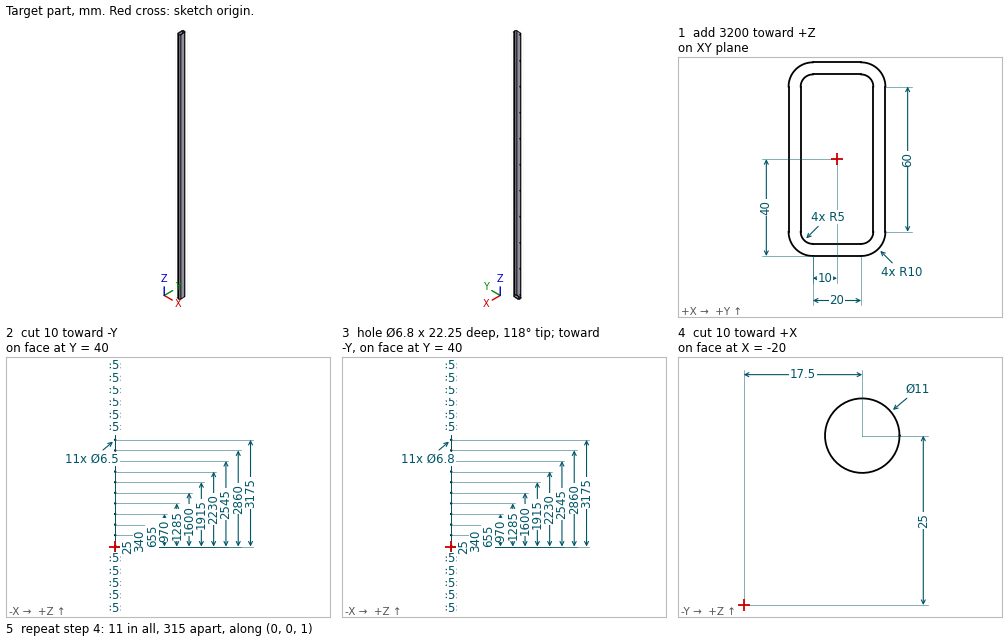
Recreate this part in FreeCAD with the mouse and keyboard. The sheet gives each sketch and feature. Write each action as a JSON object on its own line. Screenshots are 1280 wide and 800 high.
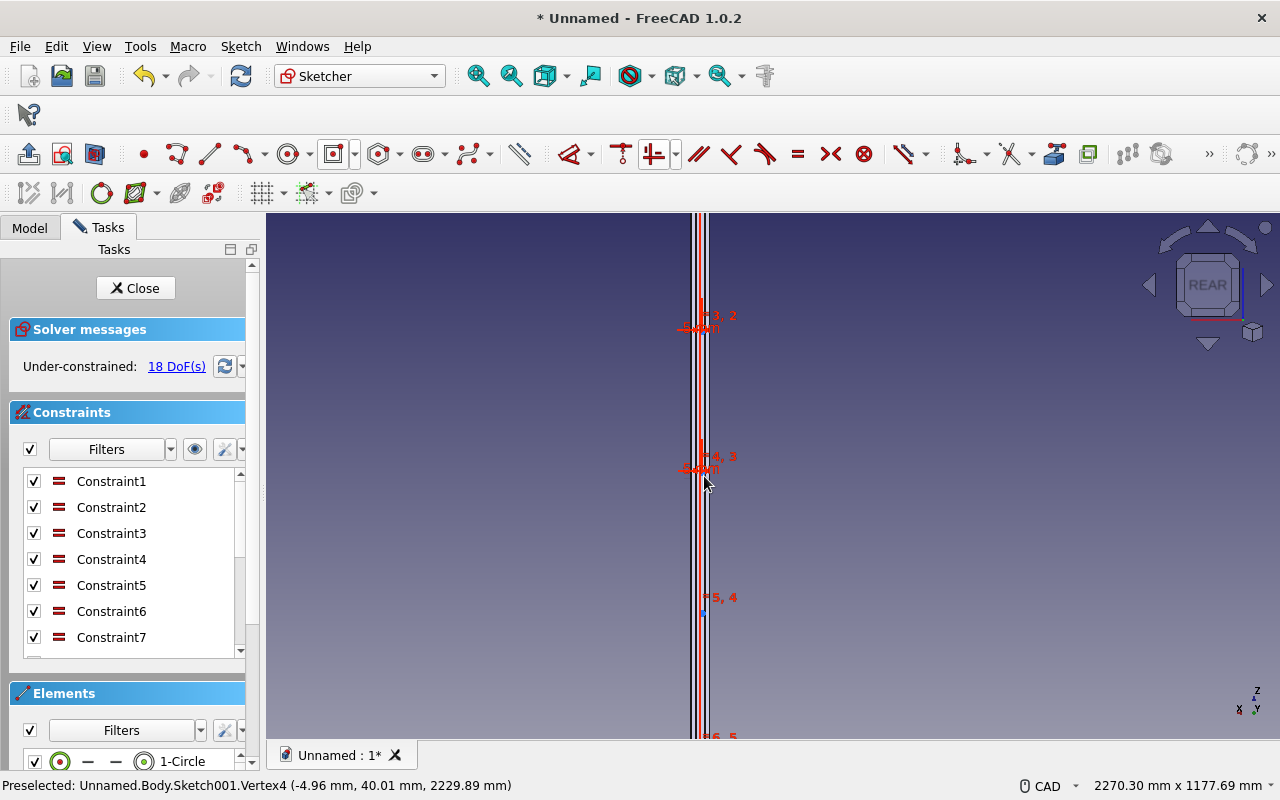
{"action": "scroll", "coordinate": [705, 383], "scroll_direction": "down", "scroll_amount": 7}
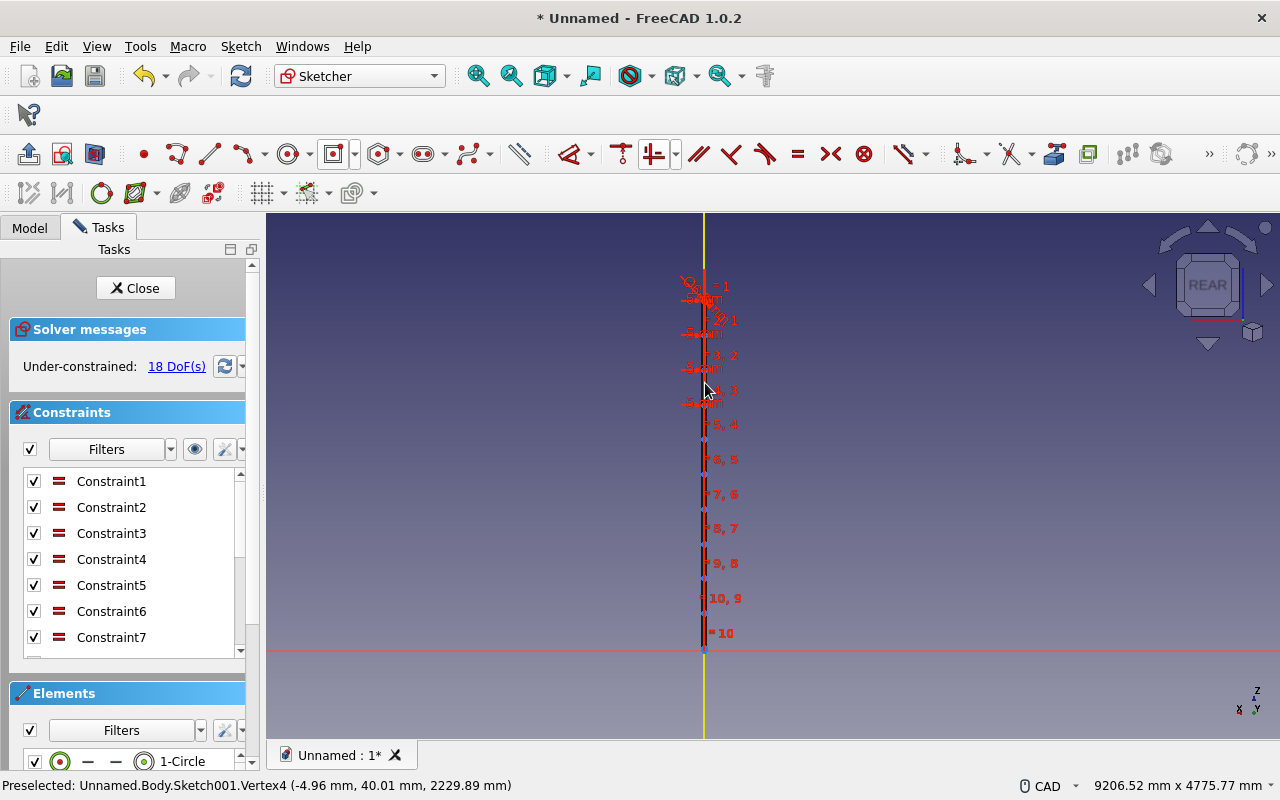
{"action": "scroll", "coordinate": [705, 440], "scroll_direction": "up", "scroll_amount": 22}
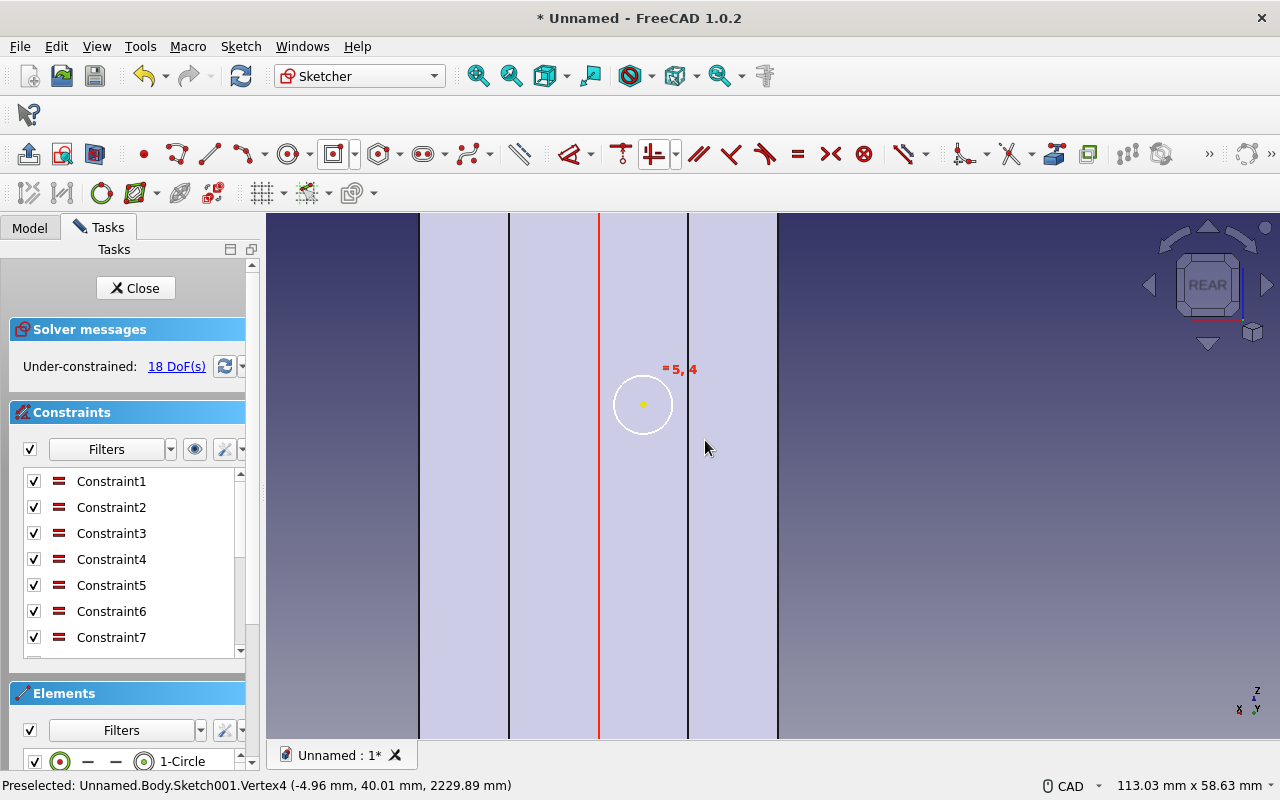
{"action": "left_click", "coordinate": [643, 405]}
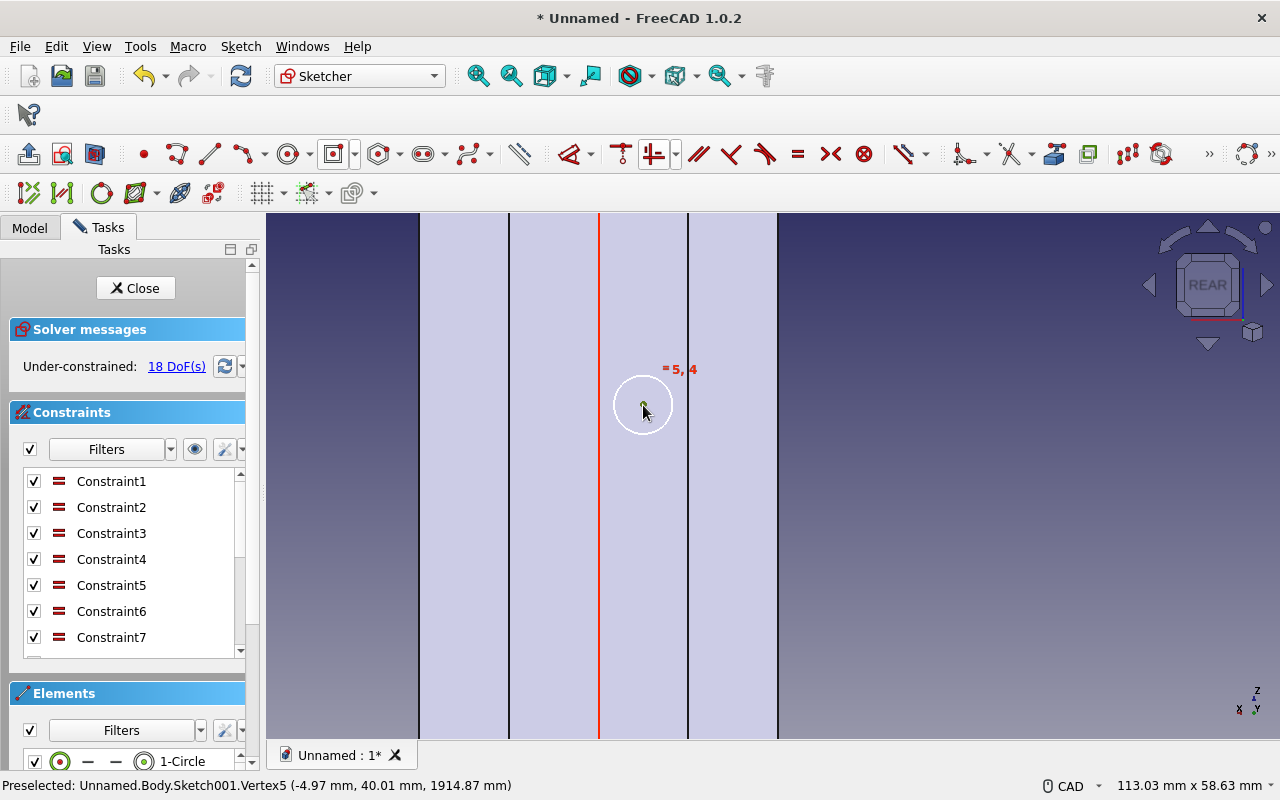
{"action": "key", "text": "l"}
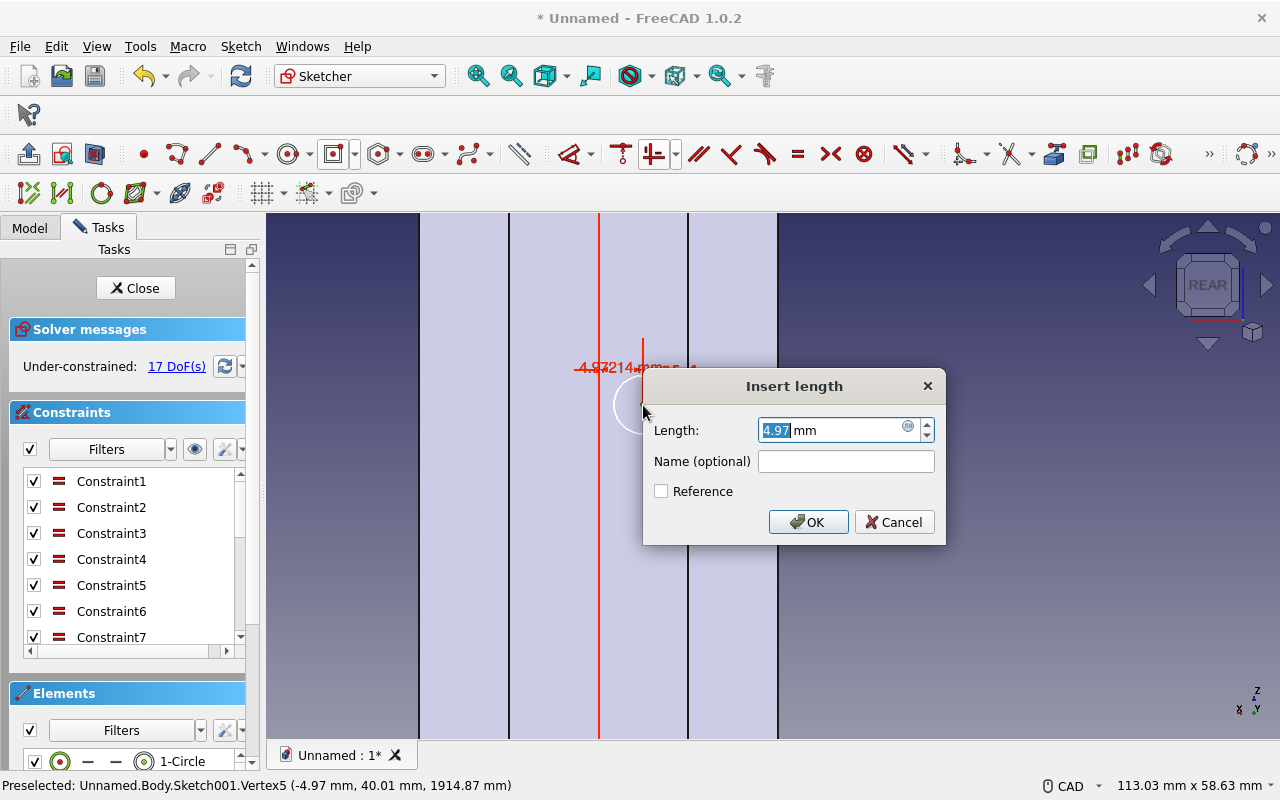
{"action": "type", "text": "5"}
{"action": "key", "text": "Return"}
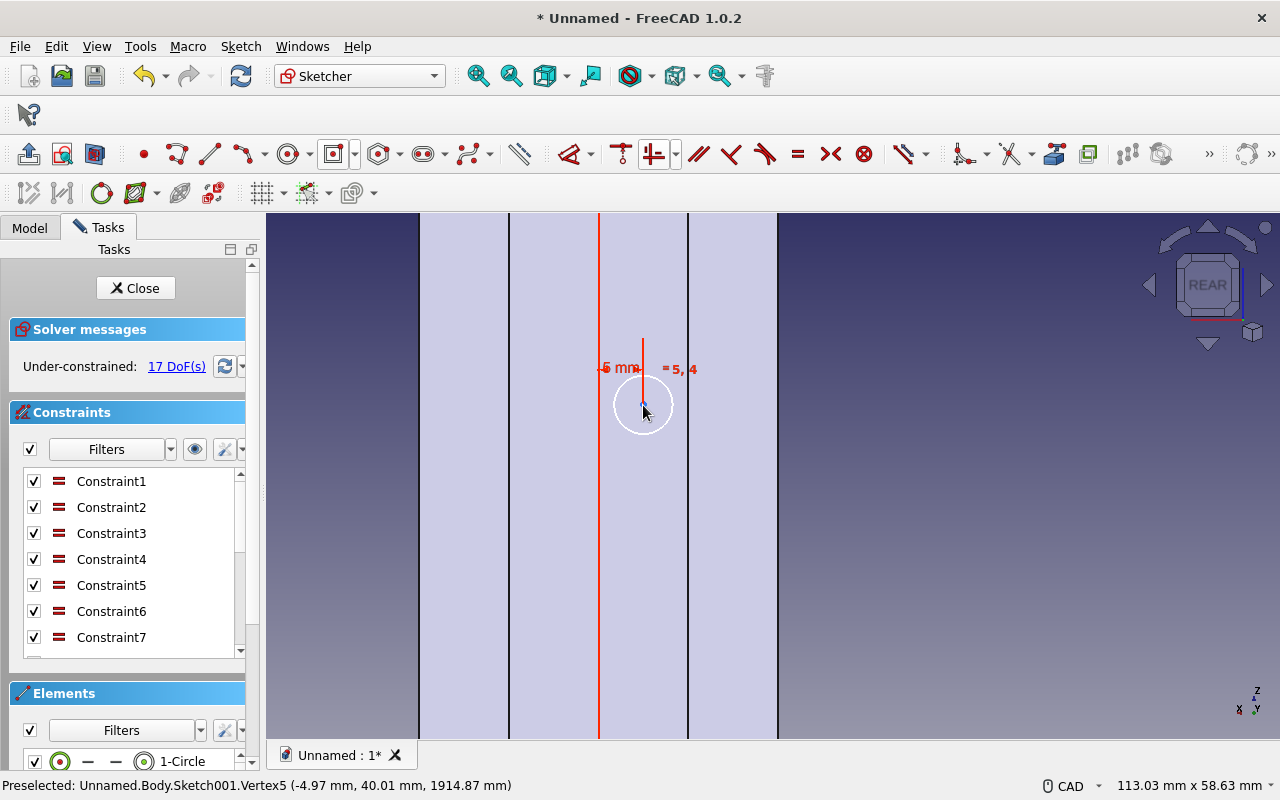
{"action": "scroll", "coordinate": [704, 476], "scroll_direction": "down", "scroll_amount": 15}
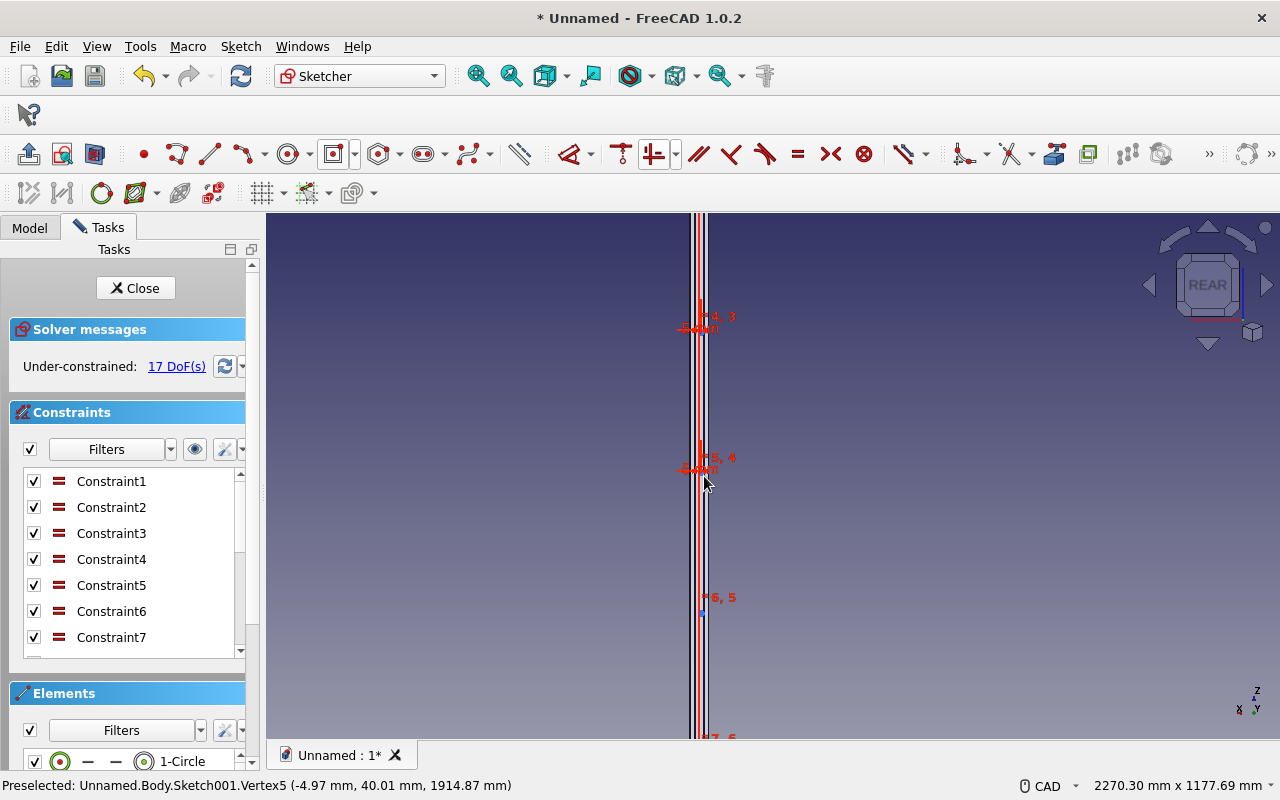
{"action": "scroll", "coordinate": [706, 429], "scroll_direction": "down", "scroll_amount": 7}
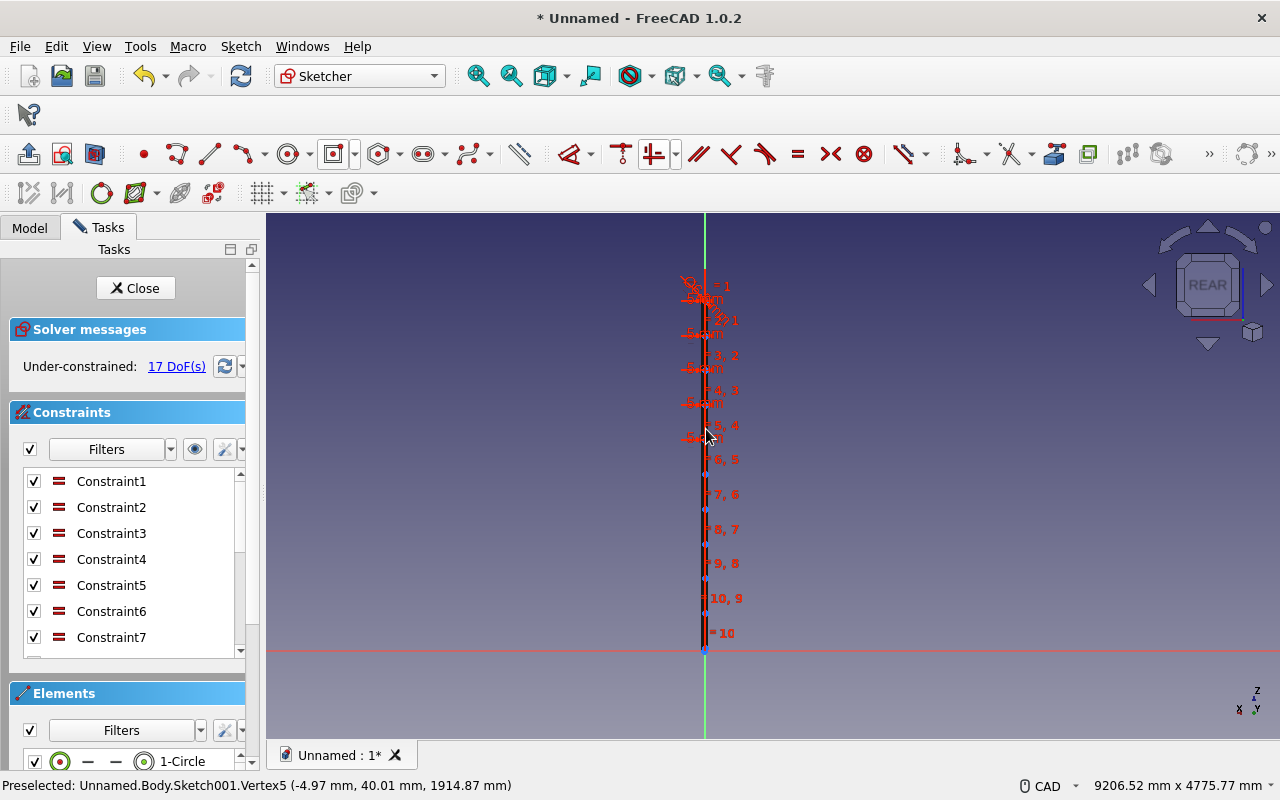
{"action": "scroll", "coordinate": [705, 475], "scroll_direction": "up", "scroll_amount": 22}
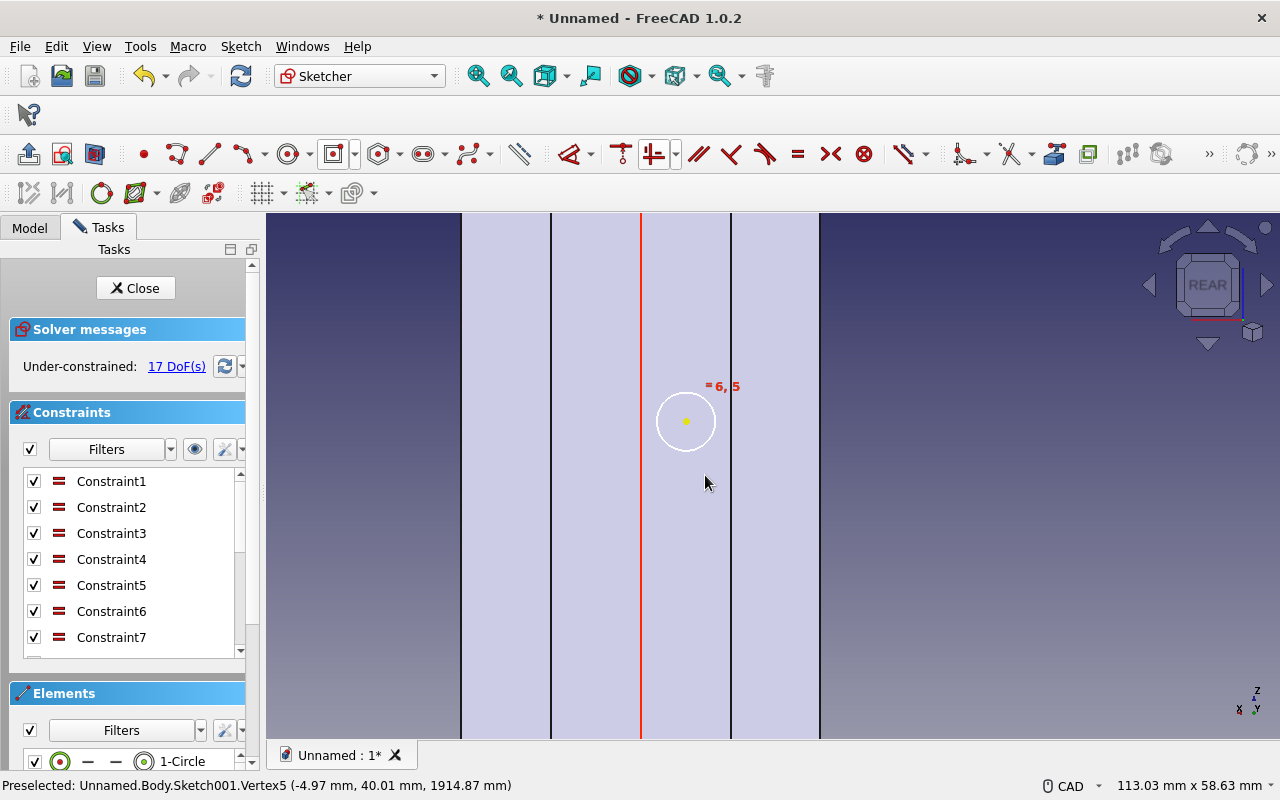
{"action": "left_click", "coordinate": [686, 422]}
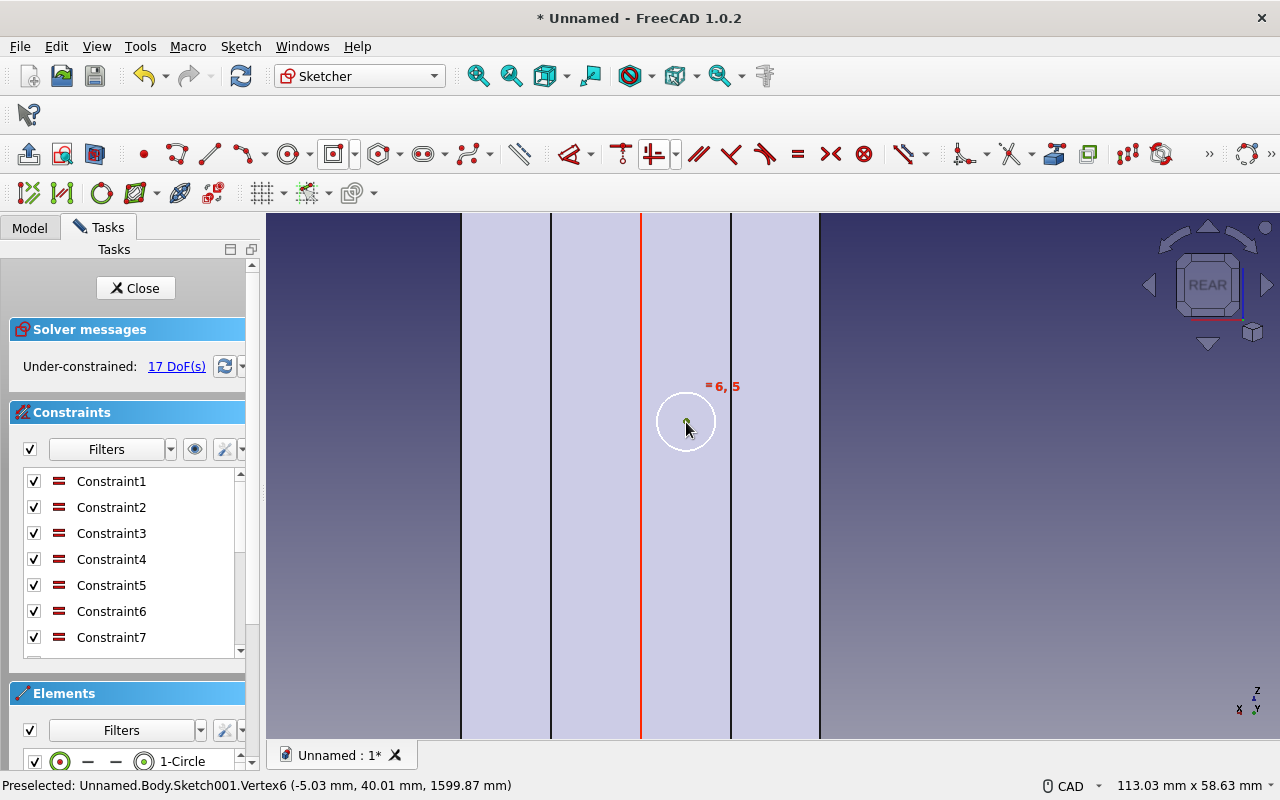
{"action": "key", "text": "l"}